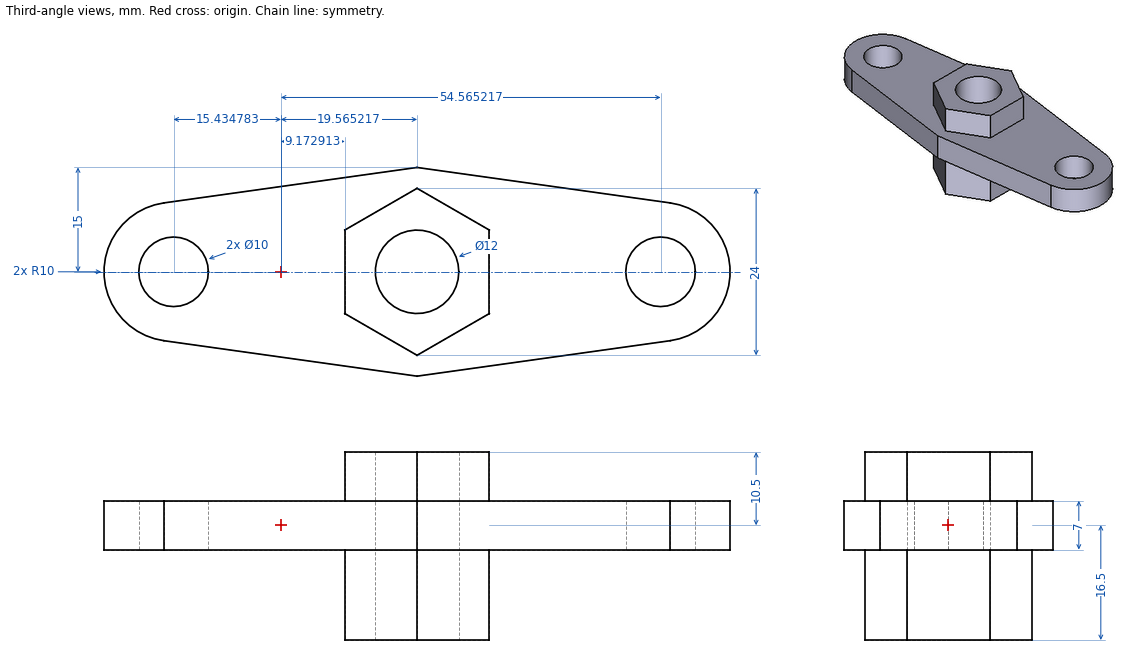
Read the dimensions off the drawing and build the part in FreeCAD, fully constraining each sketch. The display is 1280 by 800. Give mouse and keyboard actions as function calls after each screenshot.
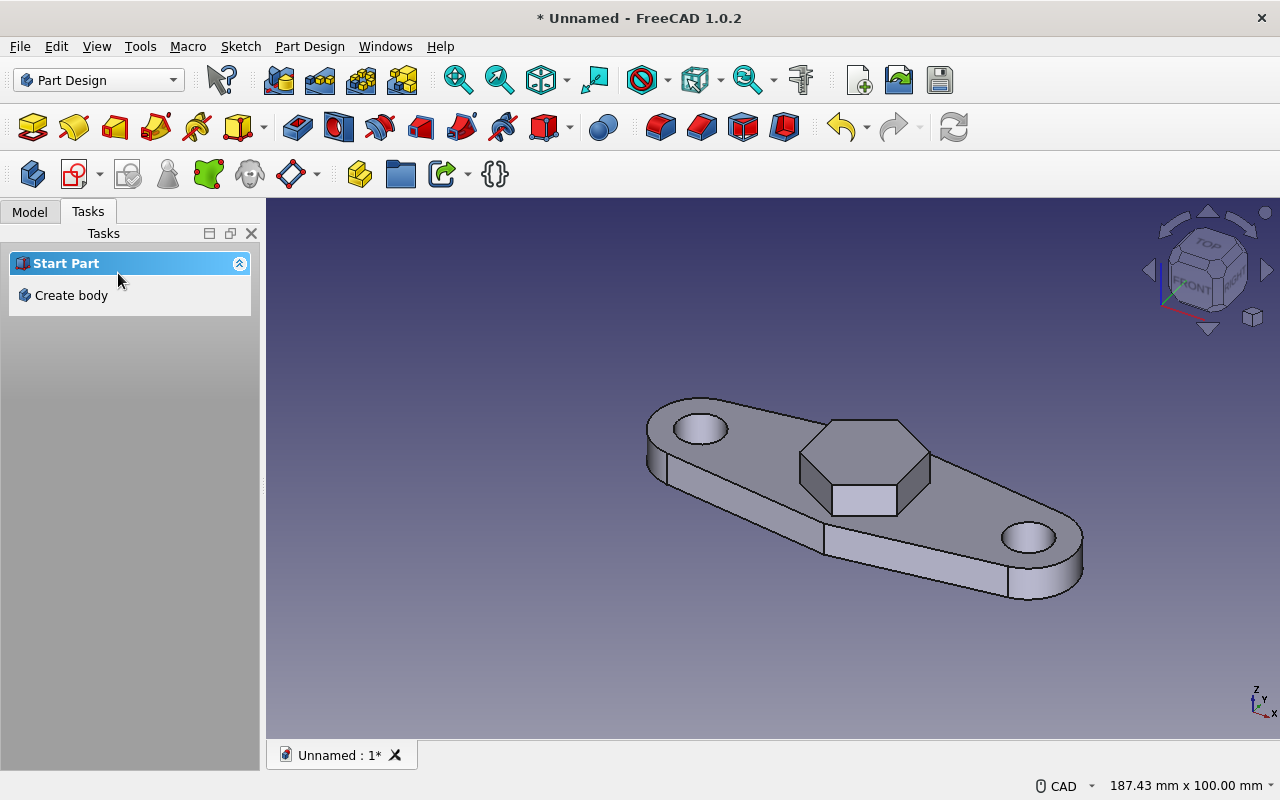
click(74, 174)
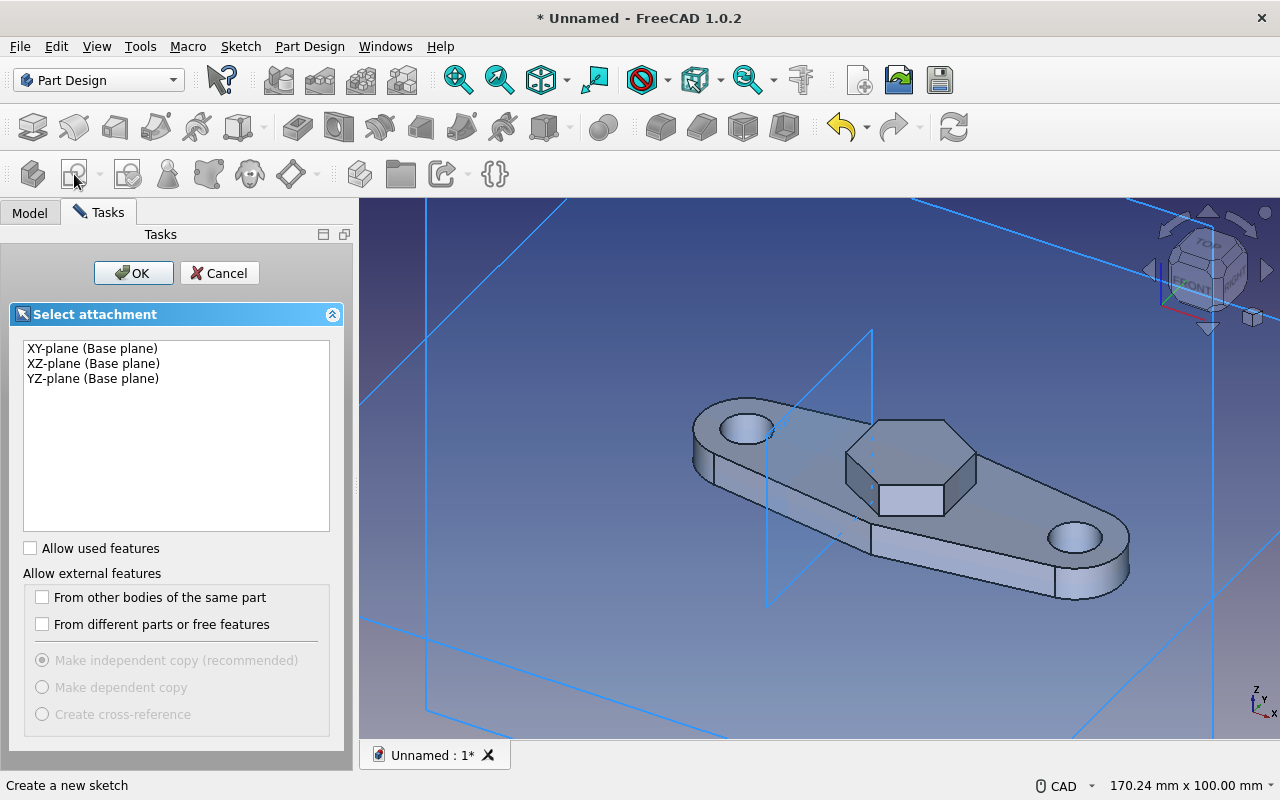
click(84, 348)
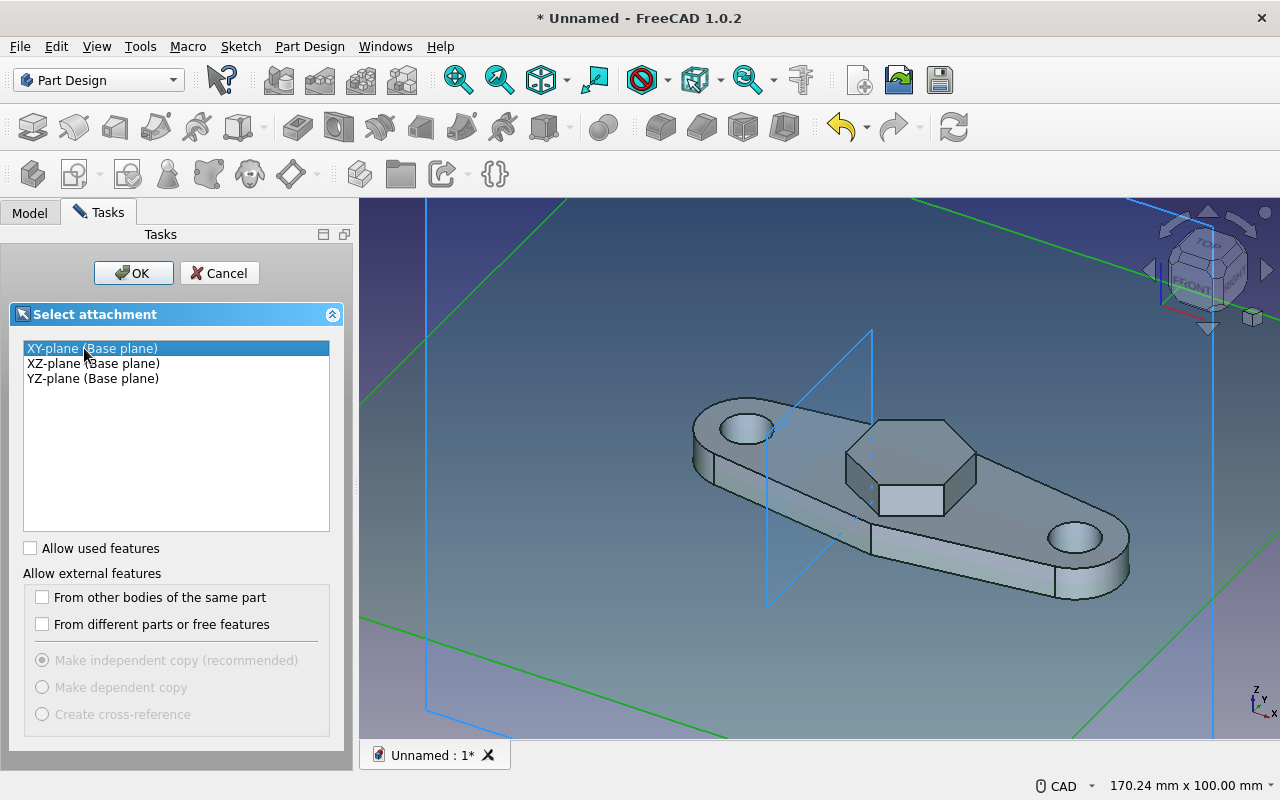
click(134, 273)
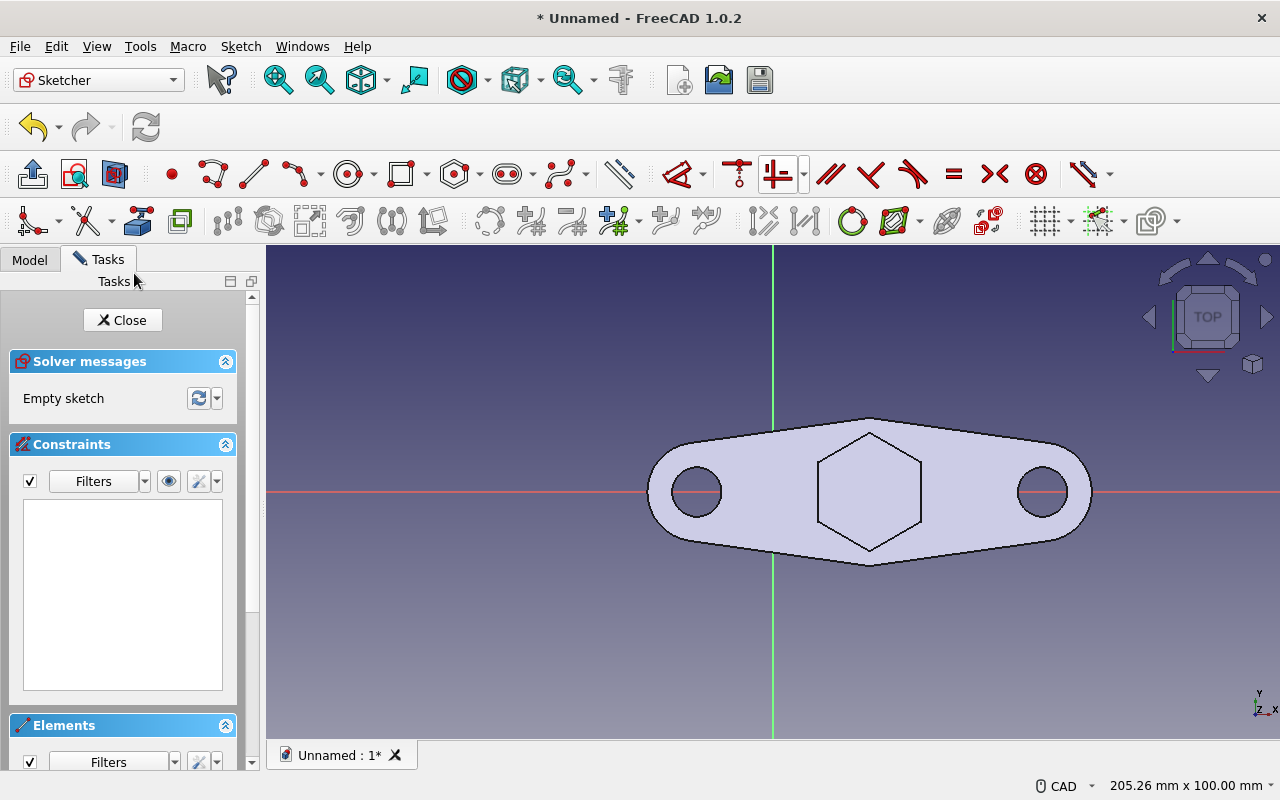
click(115, 174)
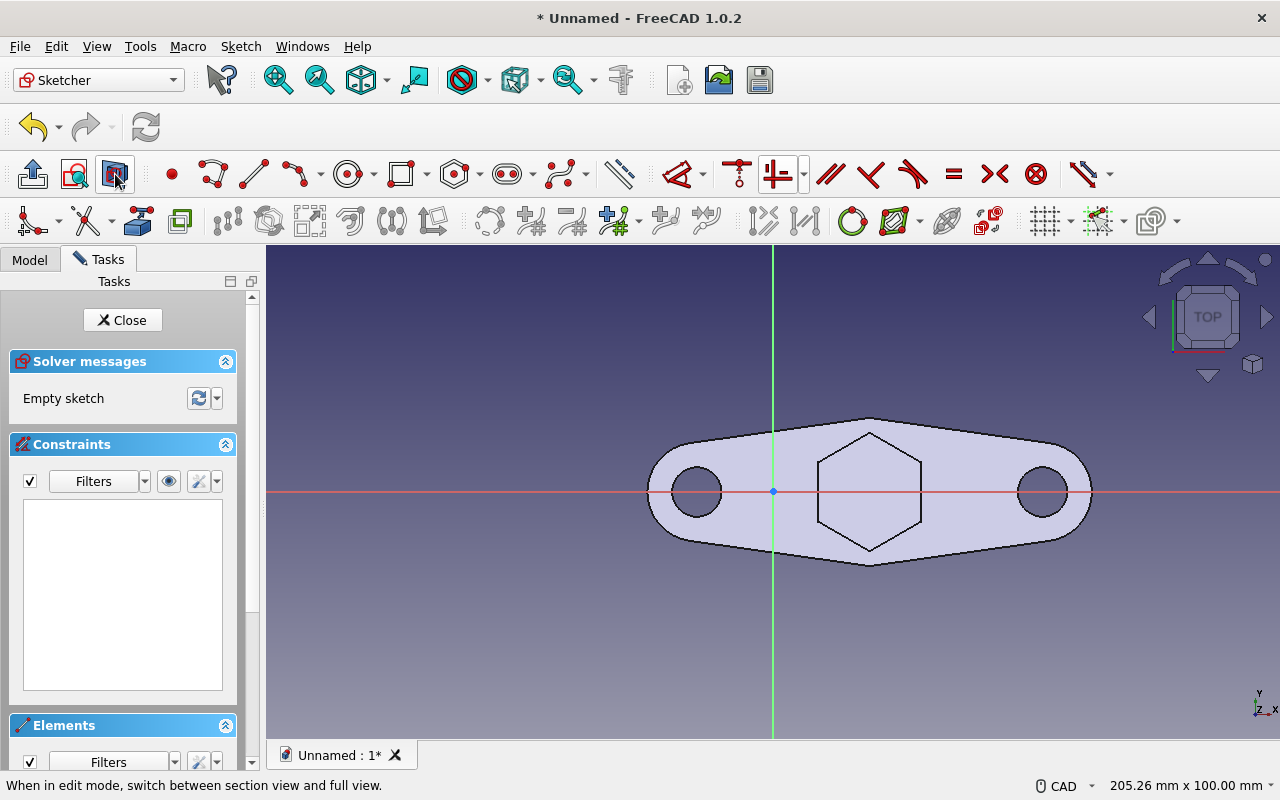
scroll(930, 492, up, 5)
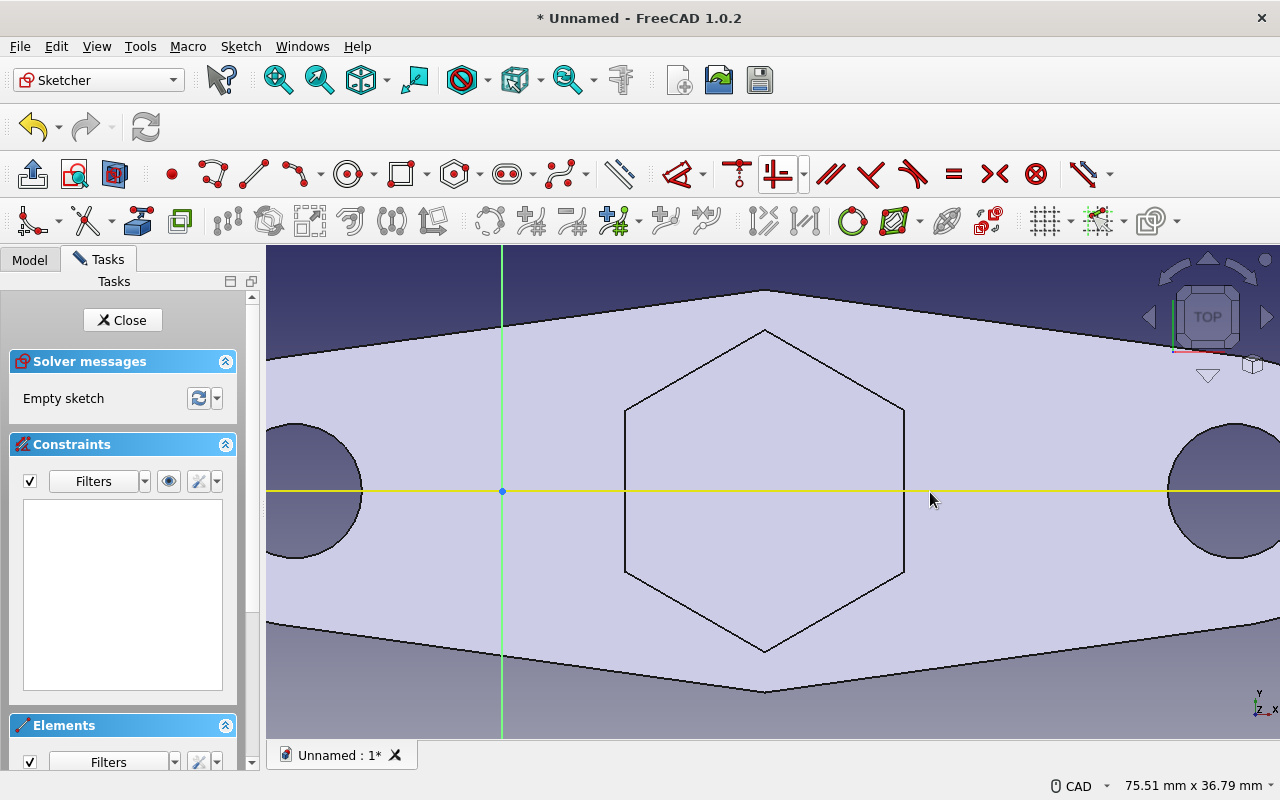
click(454, 174)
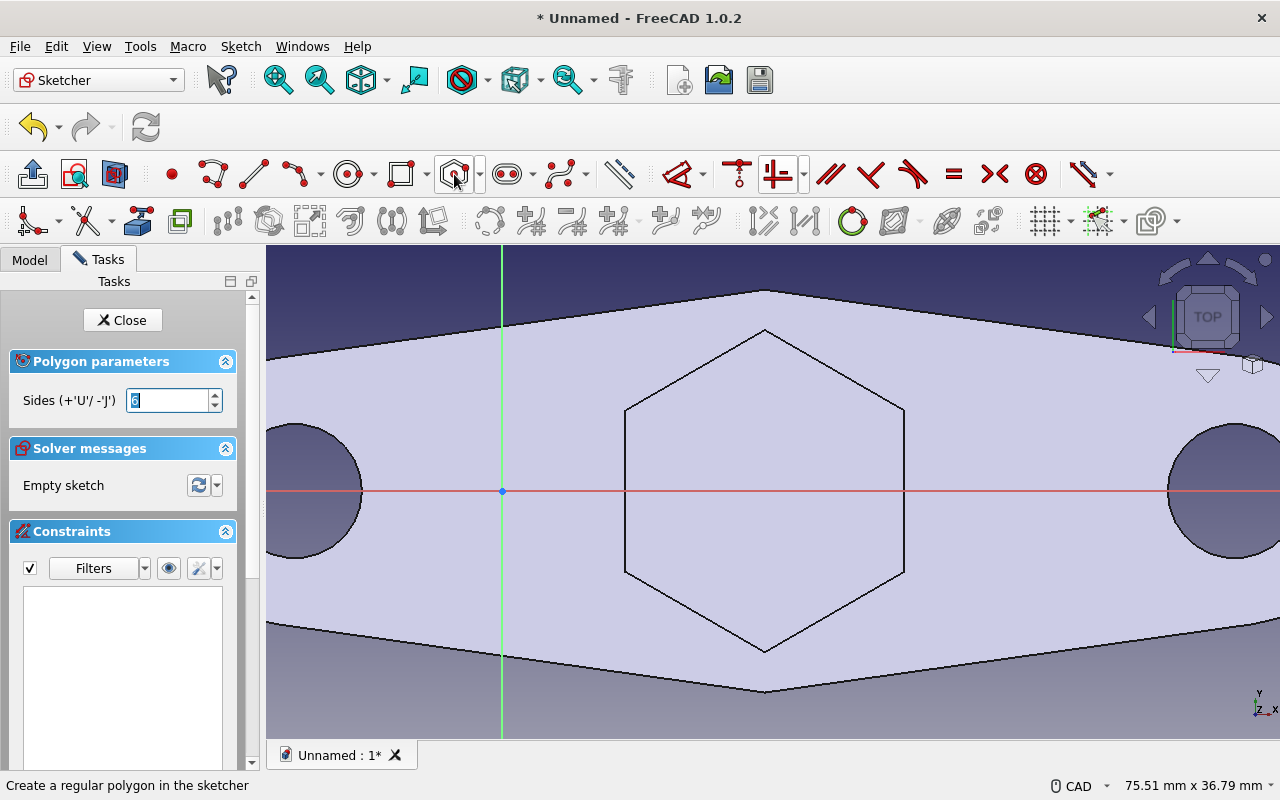
click(765, 491)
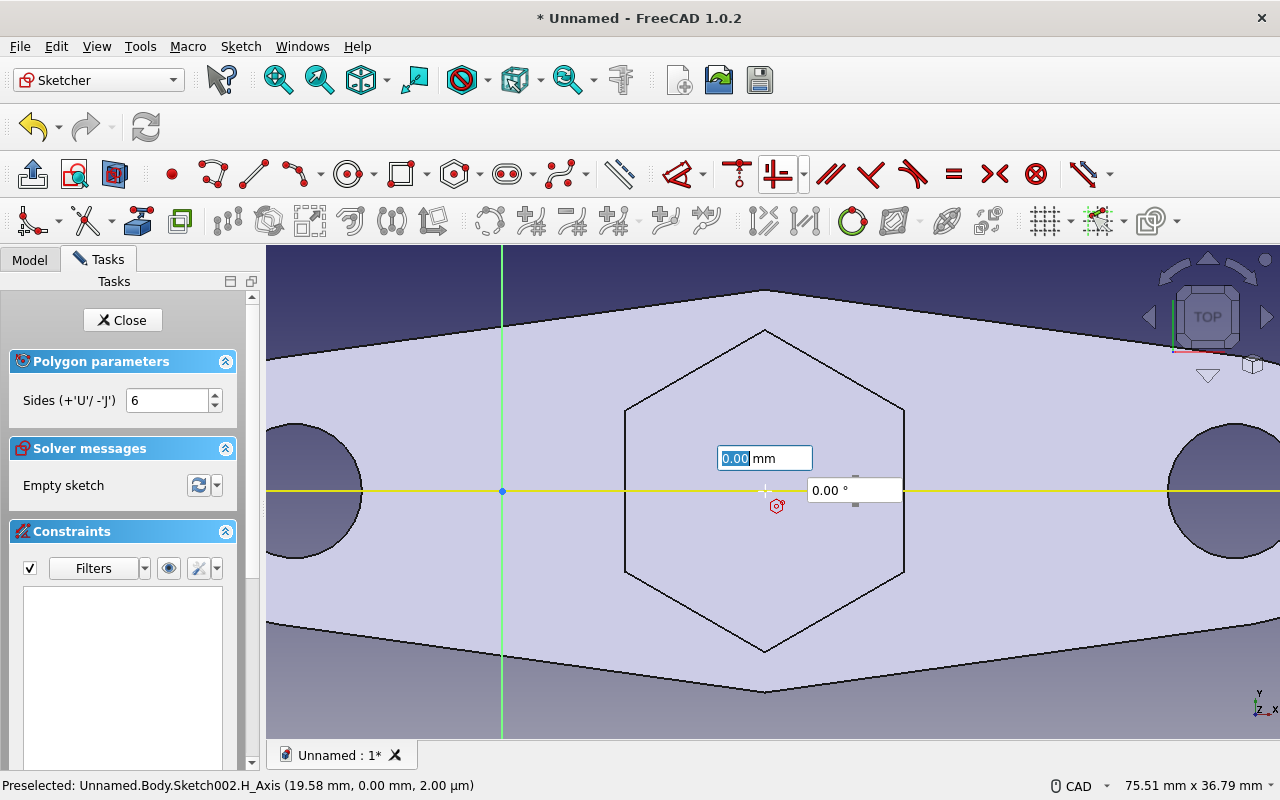
click(765, 330)
right_click(765, 330)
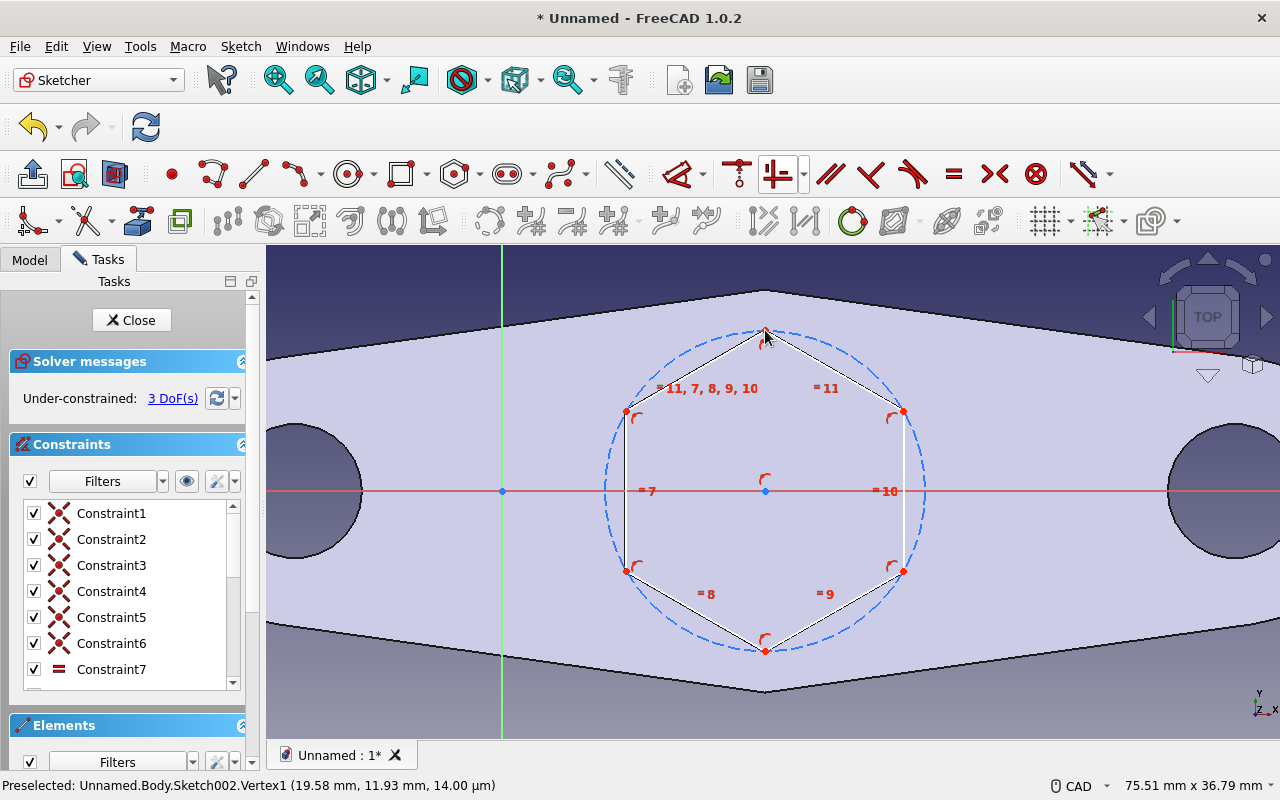
click(626, 459)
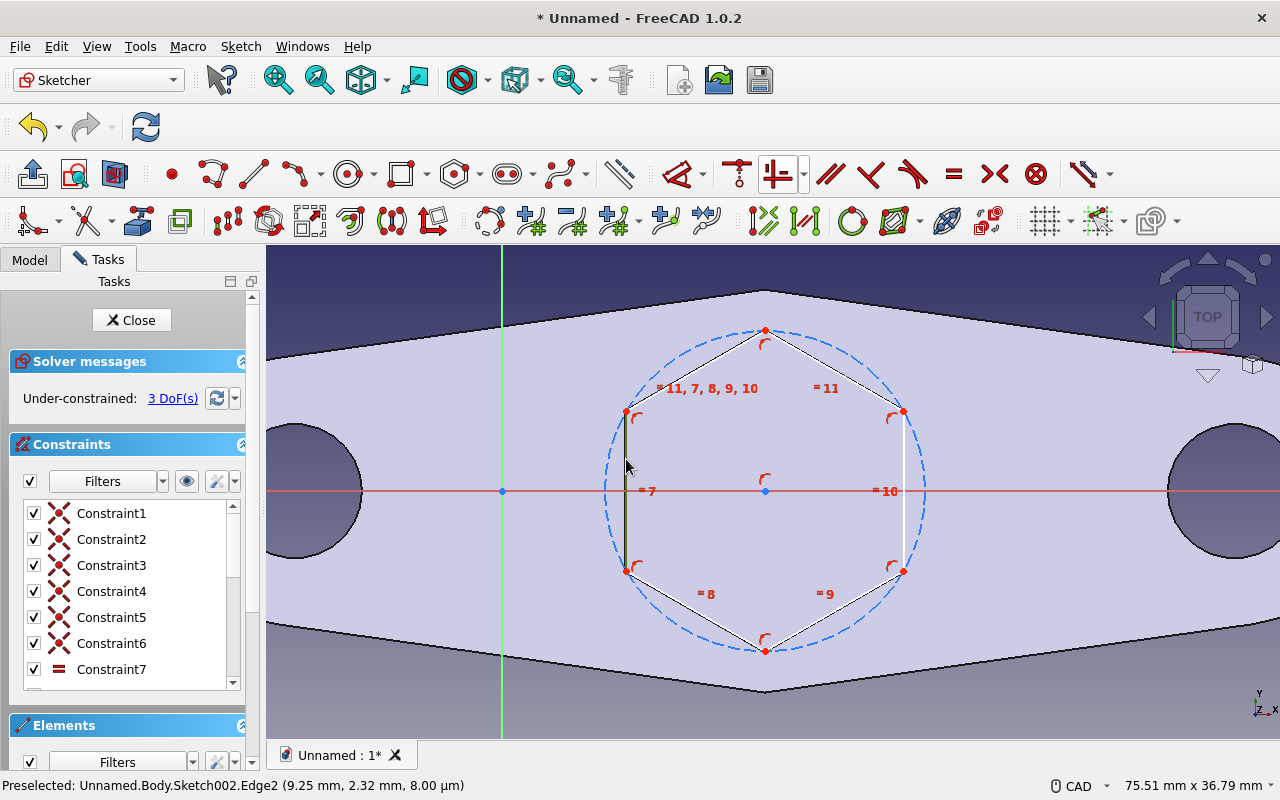
click(804, 174)